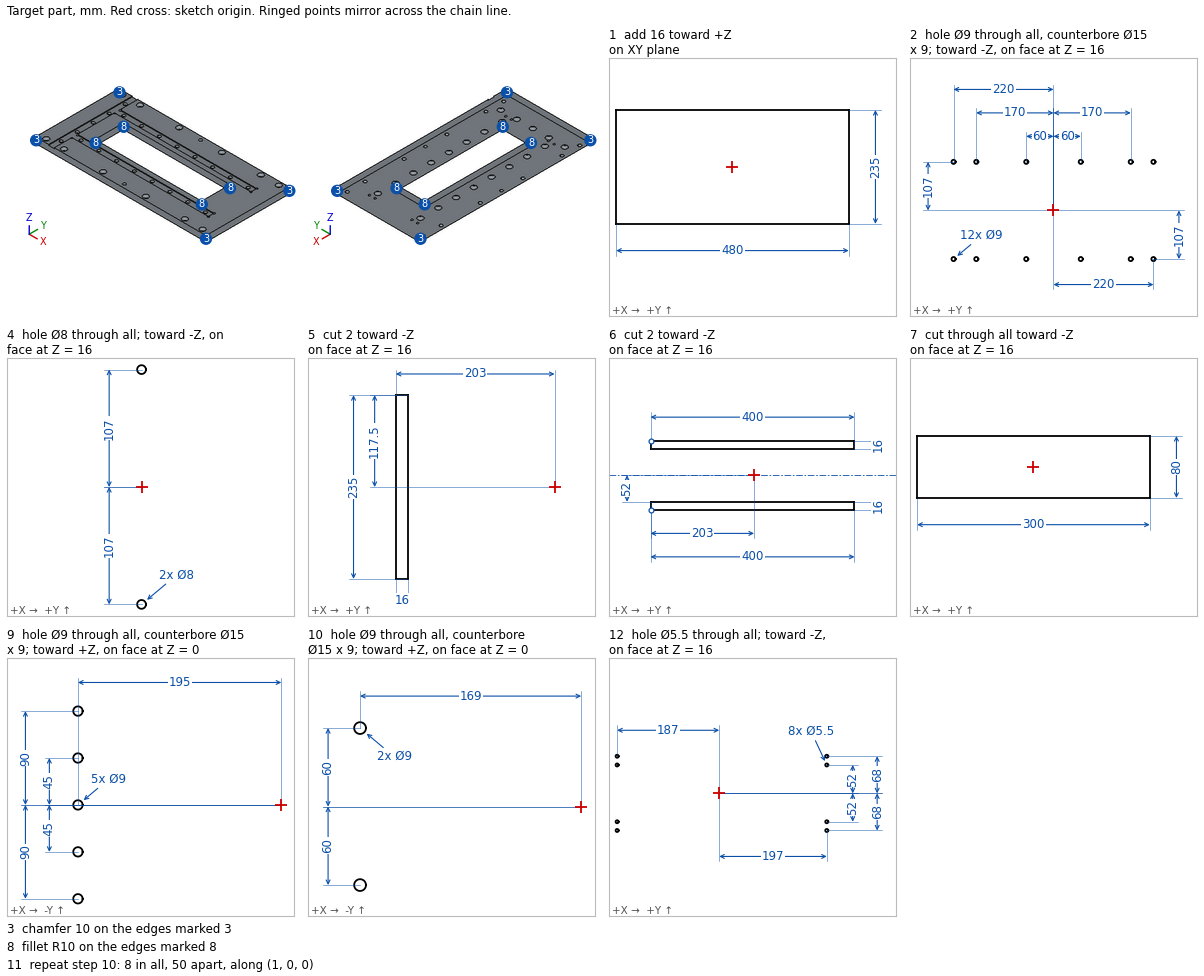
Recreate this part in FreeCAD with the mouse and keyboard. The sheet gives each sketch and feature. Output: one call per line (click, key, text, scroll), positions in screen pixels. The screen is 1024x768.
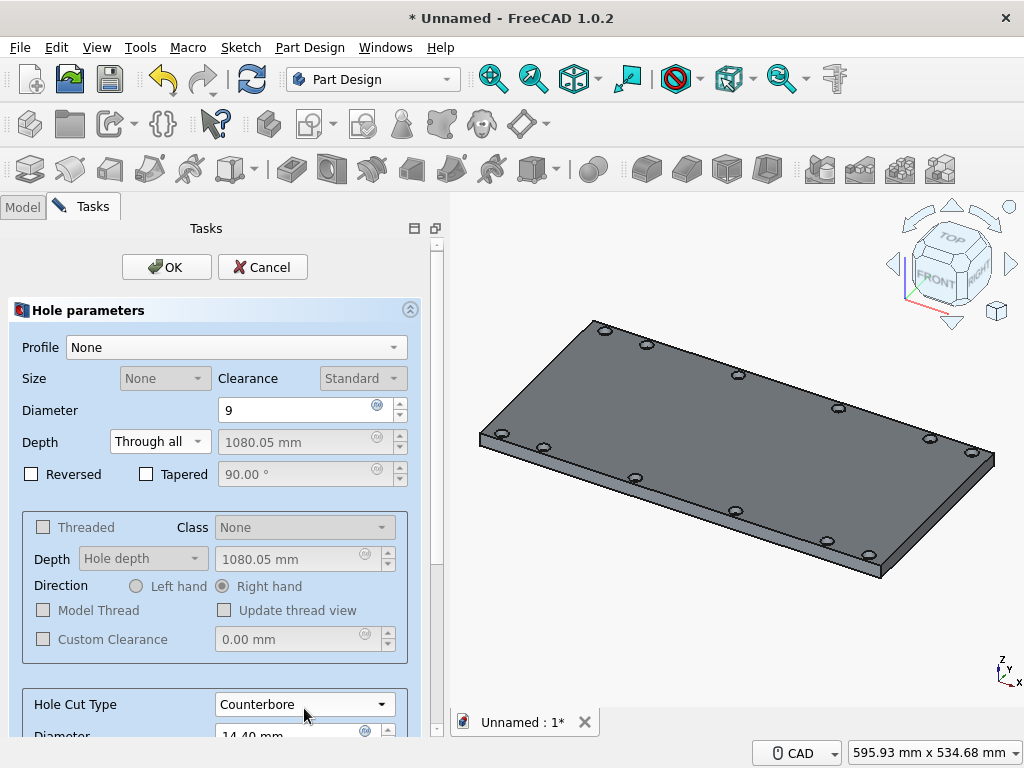
scroll(437, 487, down, 2)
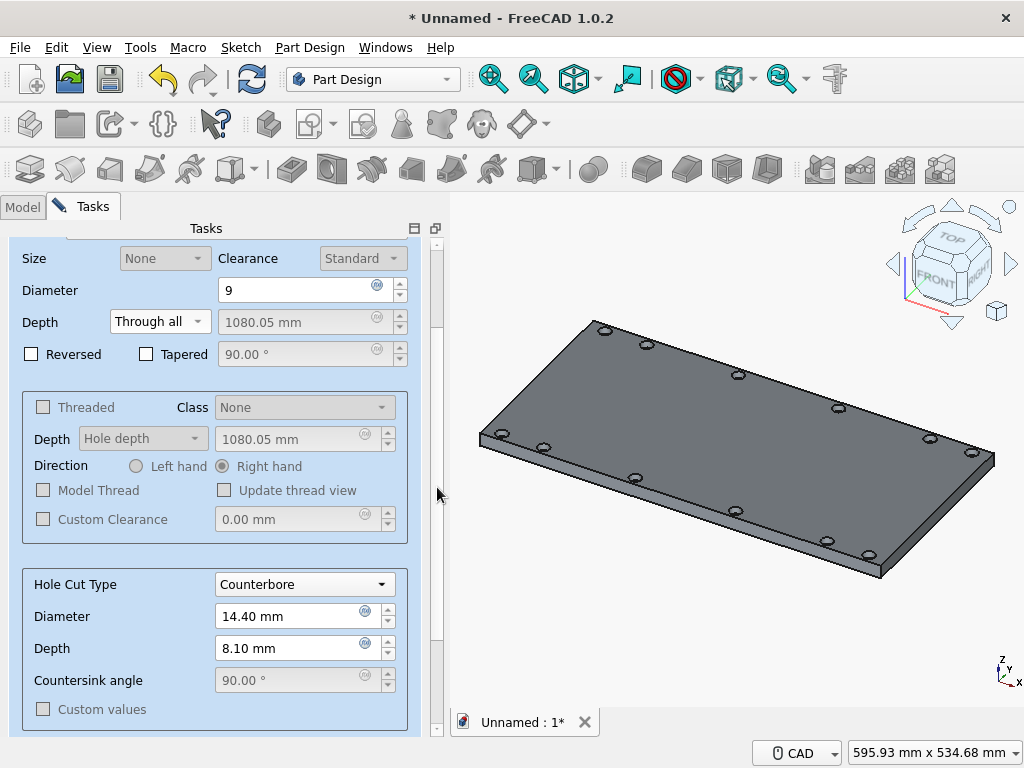
triple_click(298, 616)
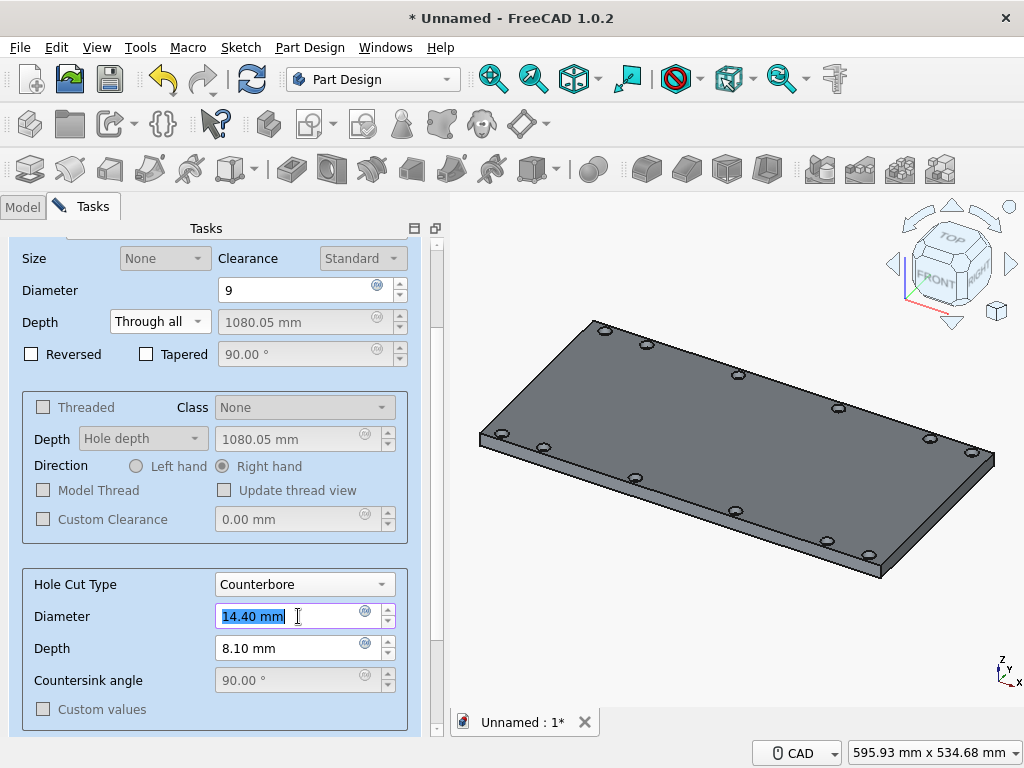
text(15)
key(Tab)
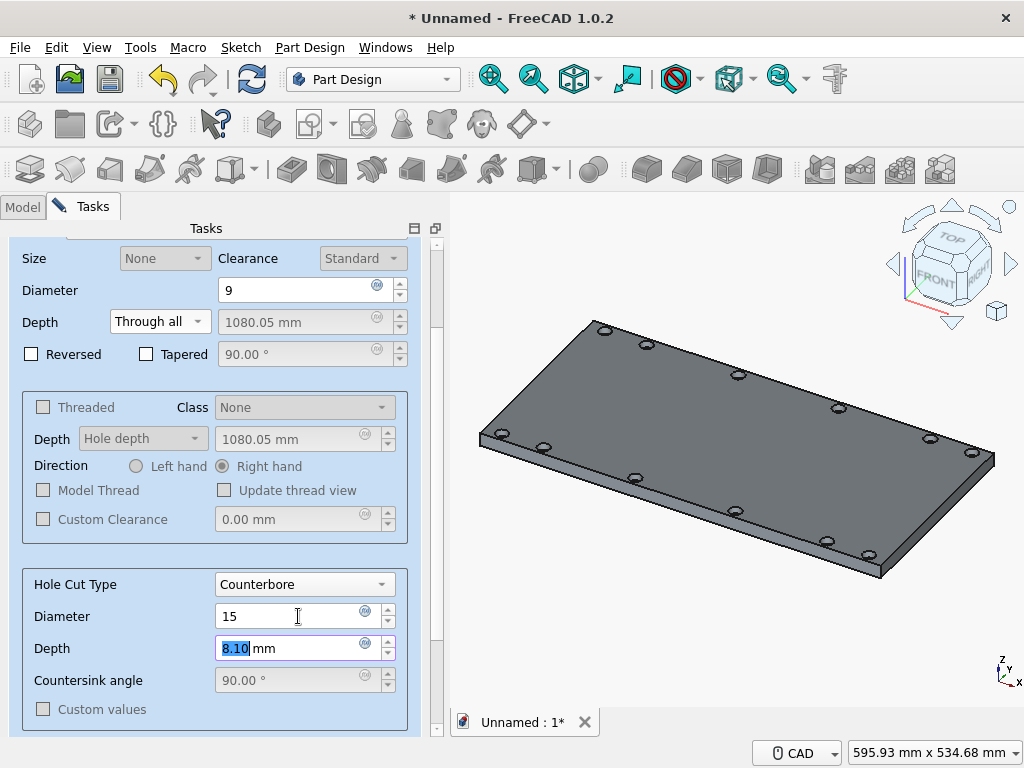
text(9)
key(Tab)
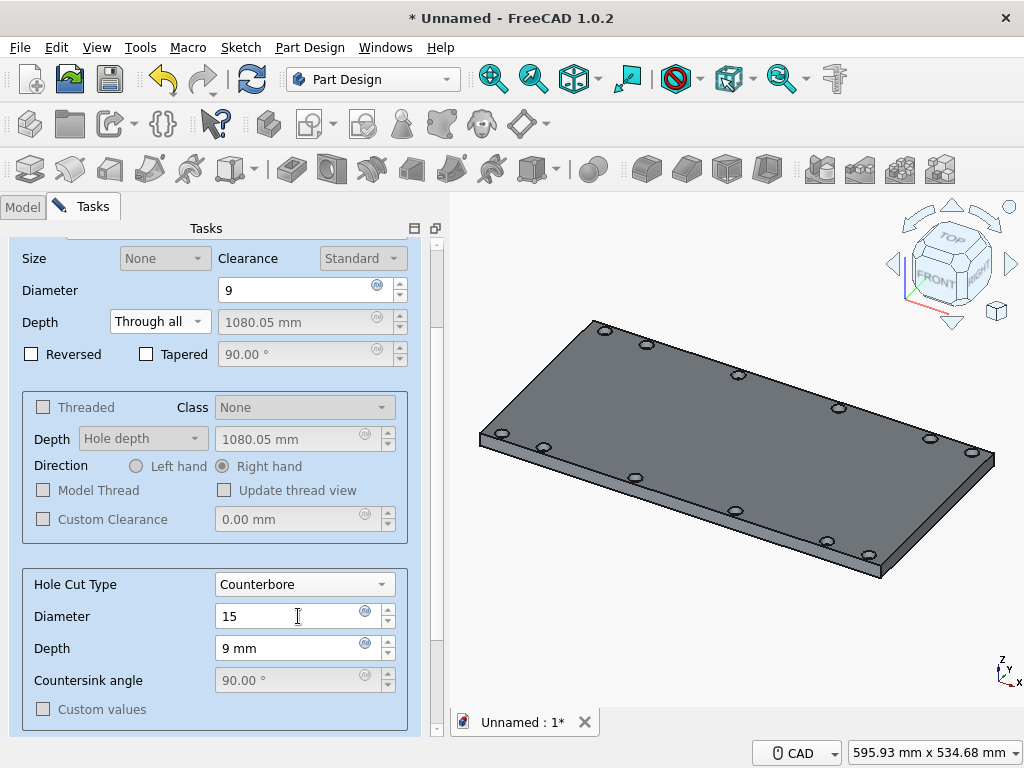
scroll(437, 487, up, 3)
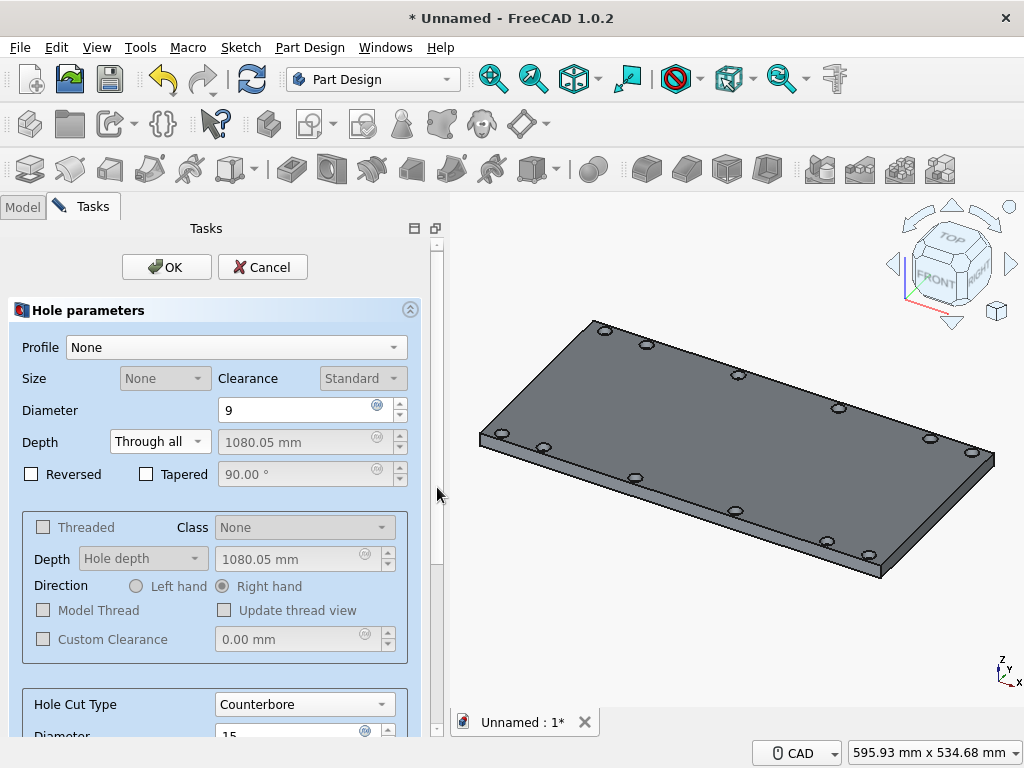
click(167, 267)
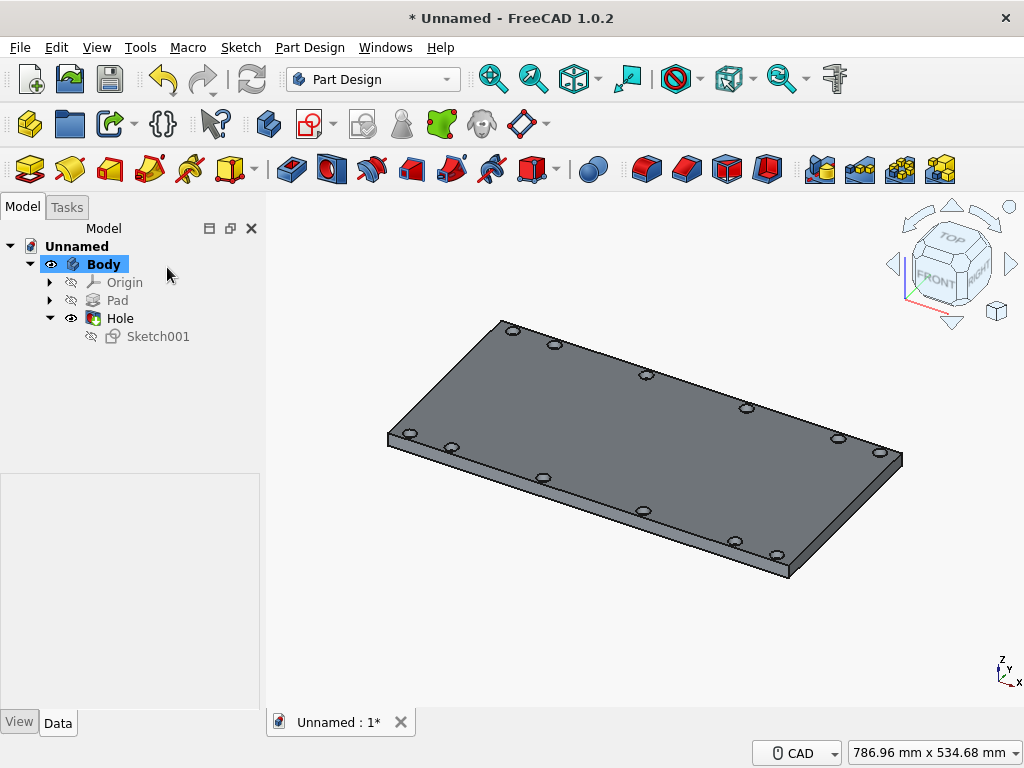
click(789, 571)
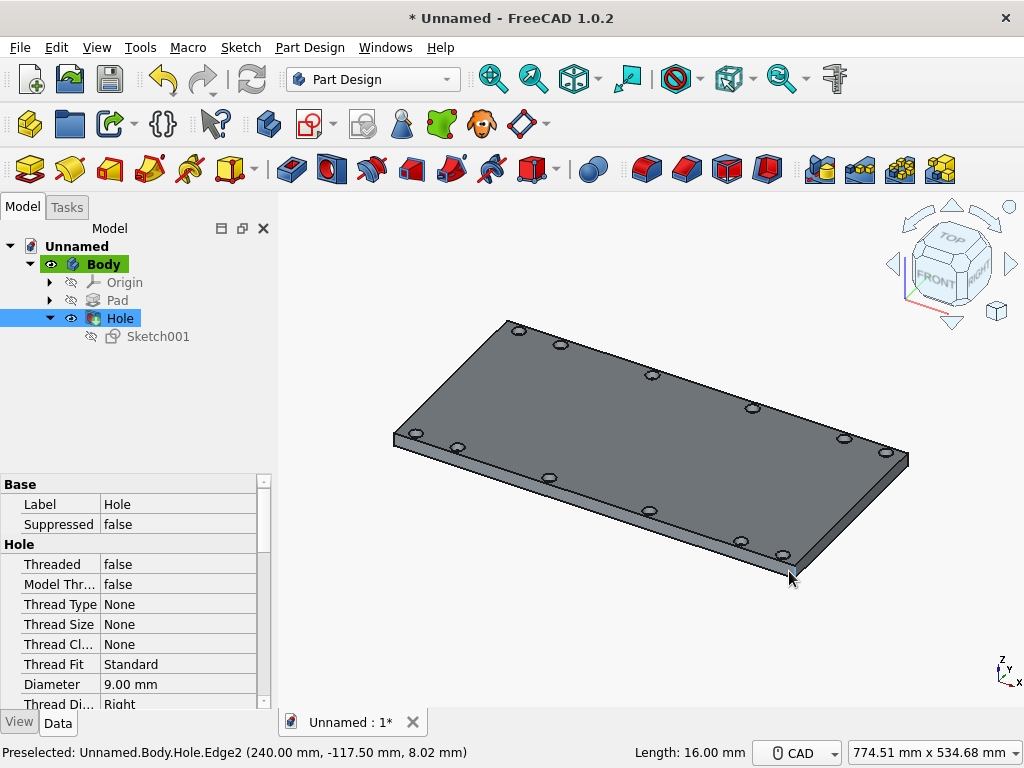
scroll(507, 326, up, 5)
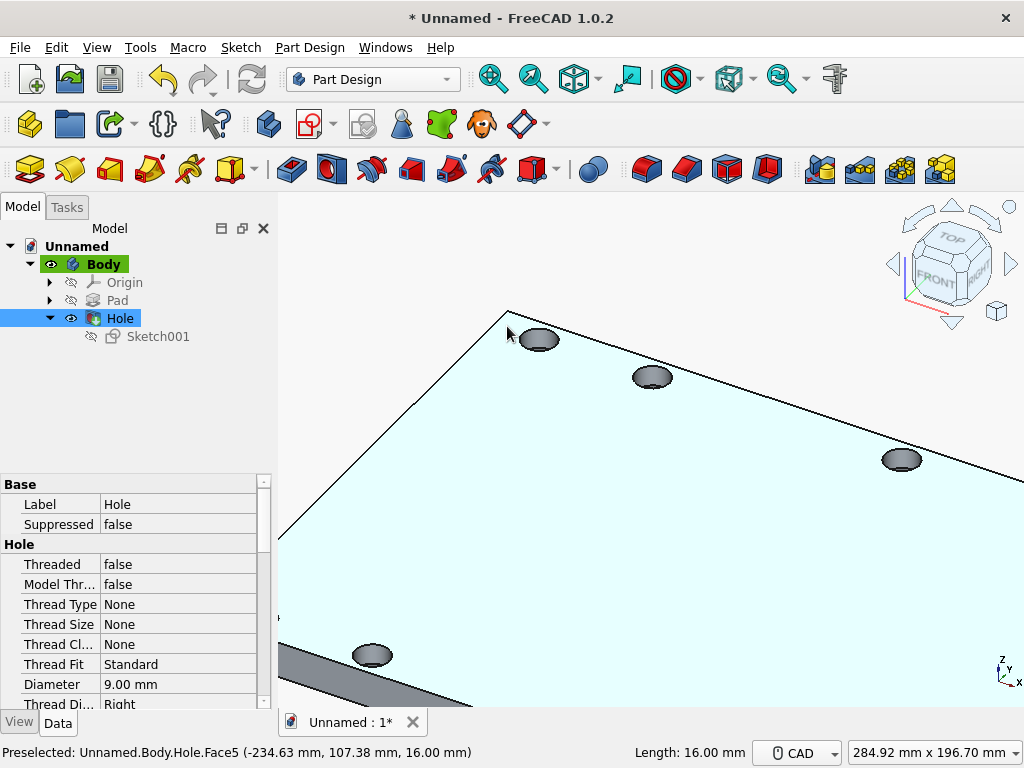
click(494, 80)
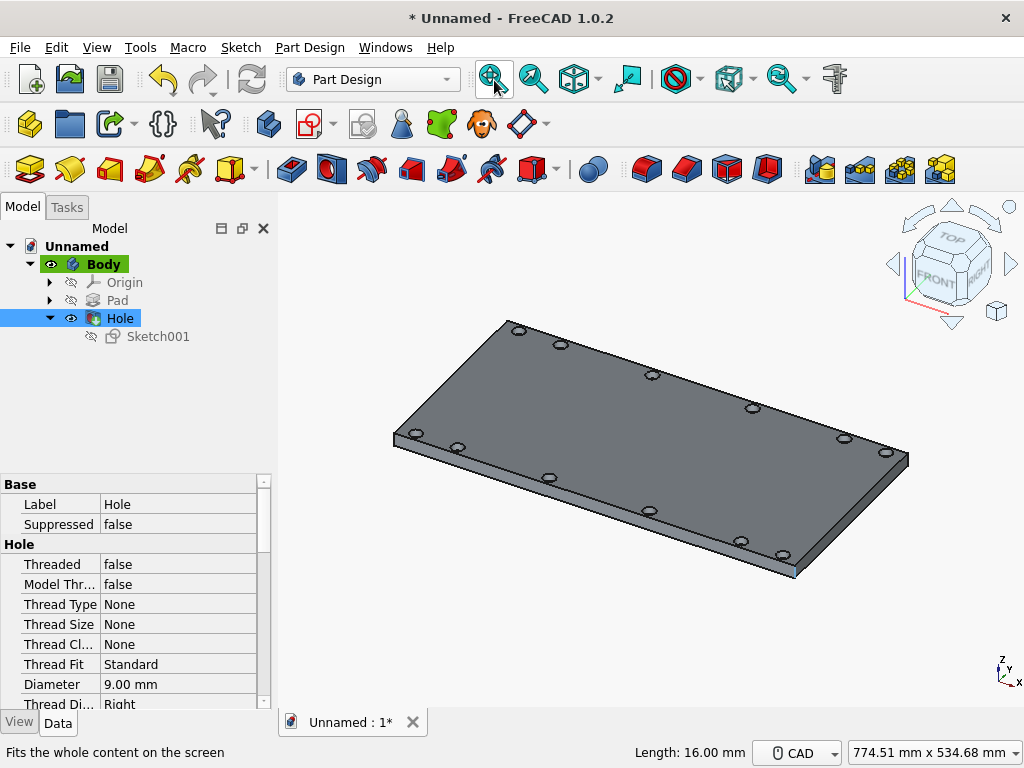
key(0)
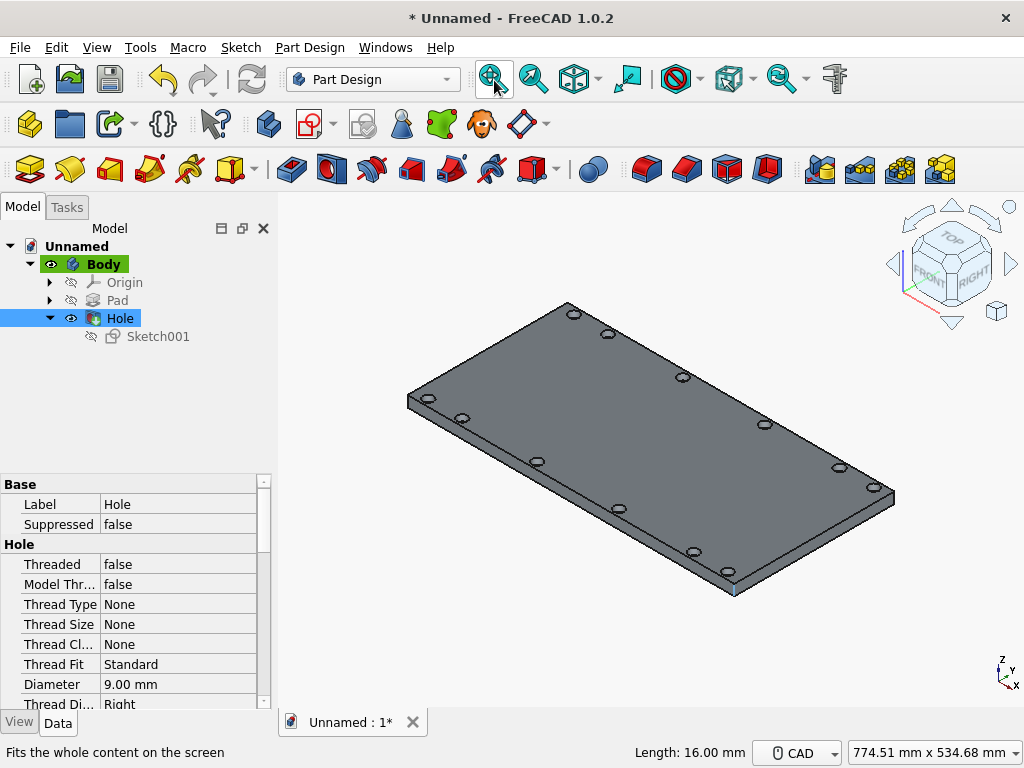
scroll(568, 308, up, 5)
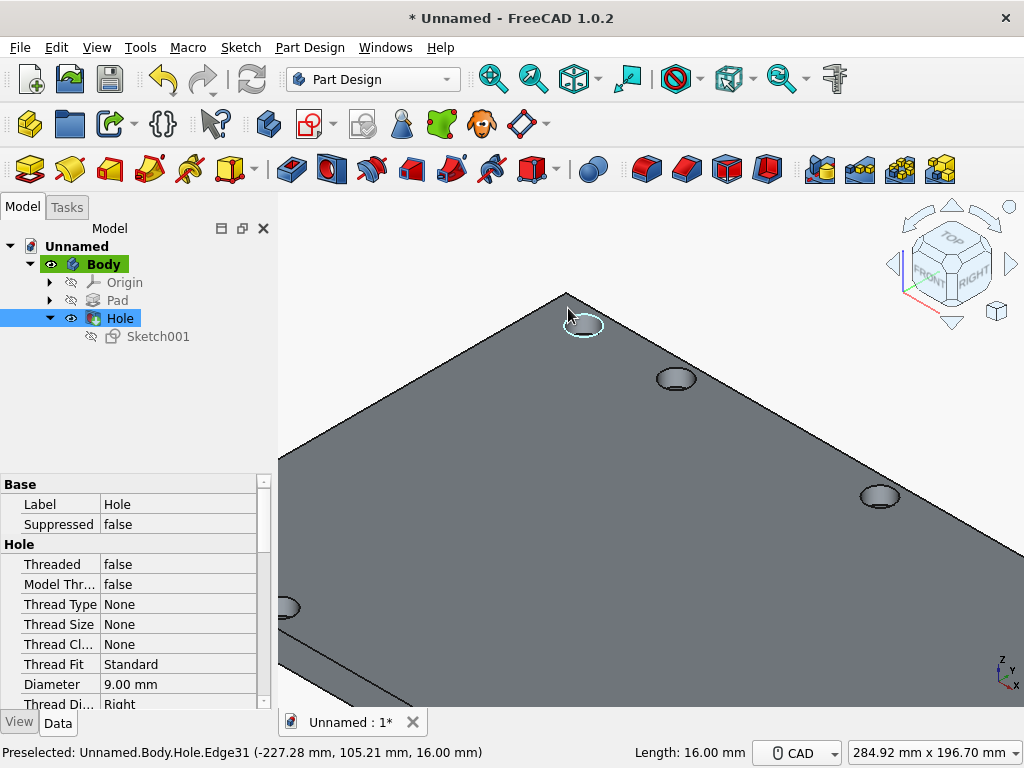
click(494, 80)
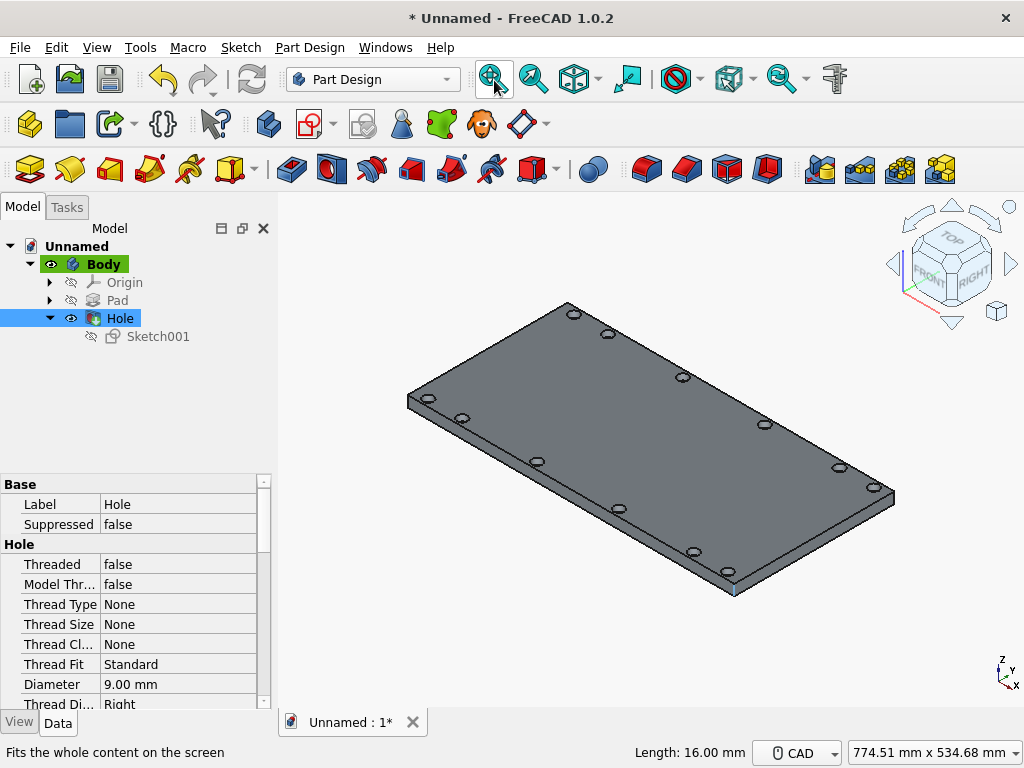
key(2)